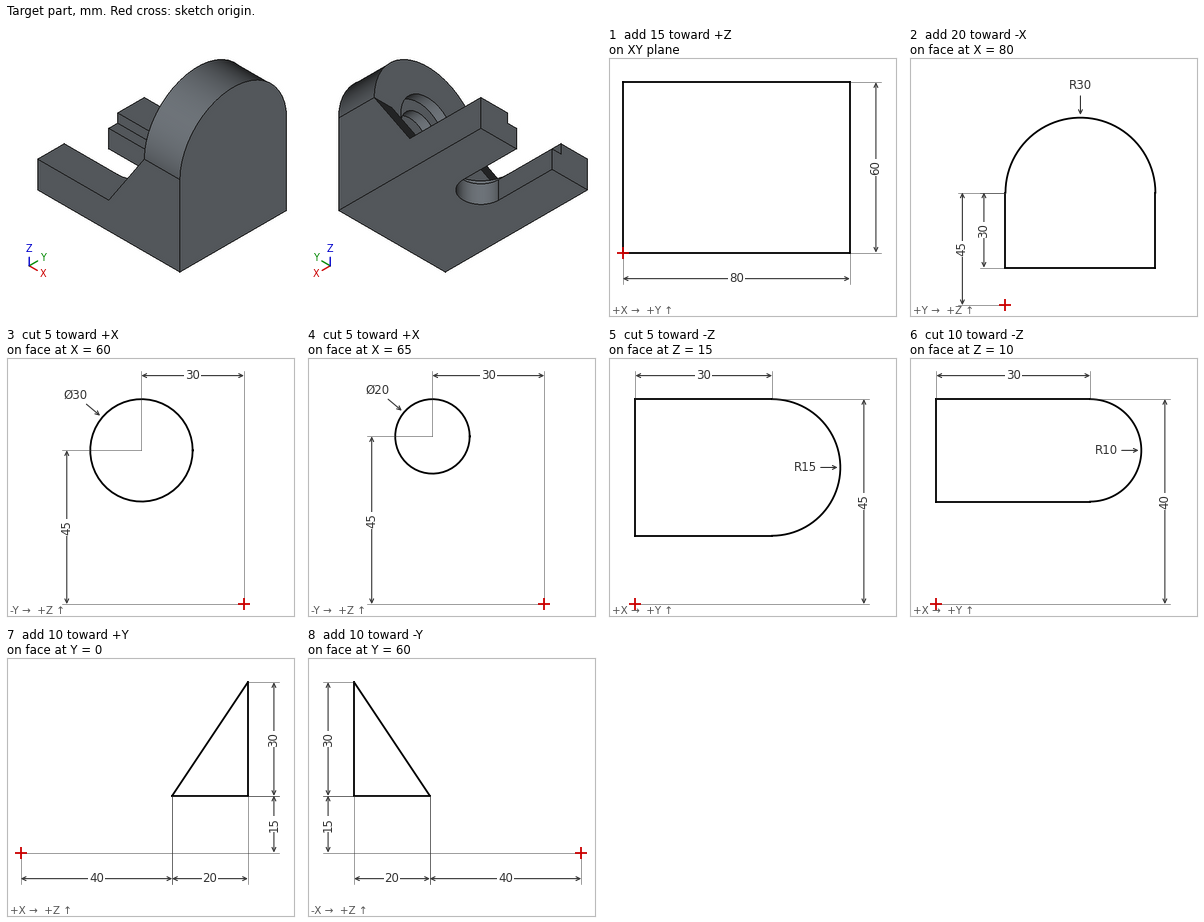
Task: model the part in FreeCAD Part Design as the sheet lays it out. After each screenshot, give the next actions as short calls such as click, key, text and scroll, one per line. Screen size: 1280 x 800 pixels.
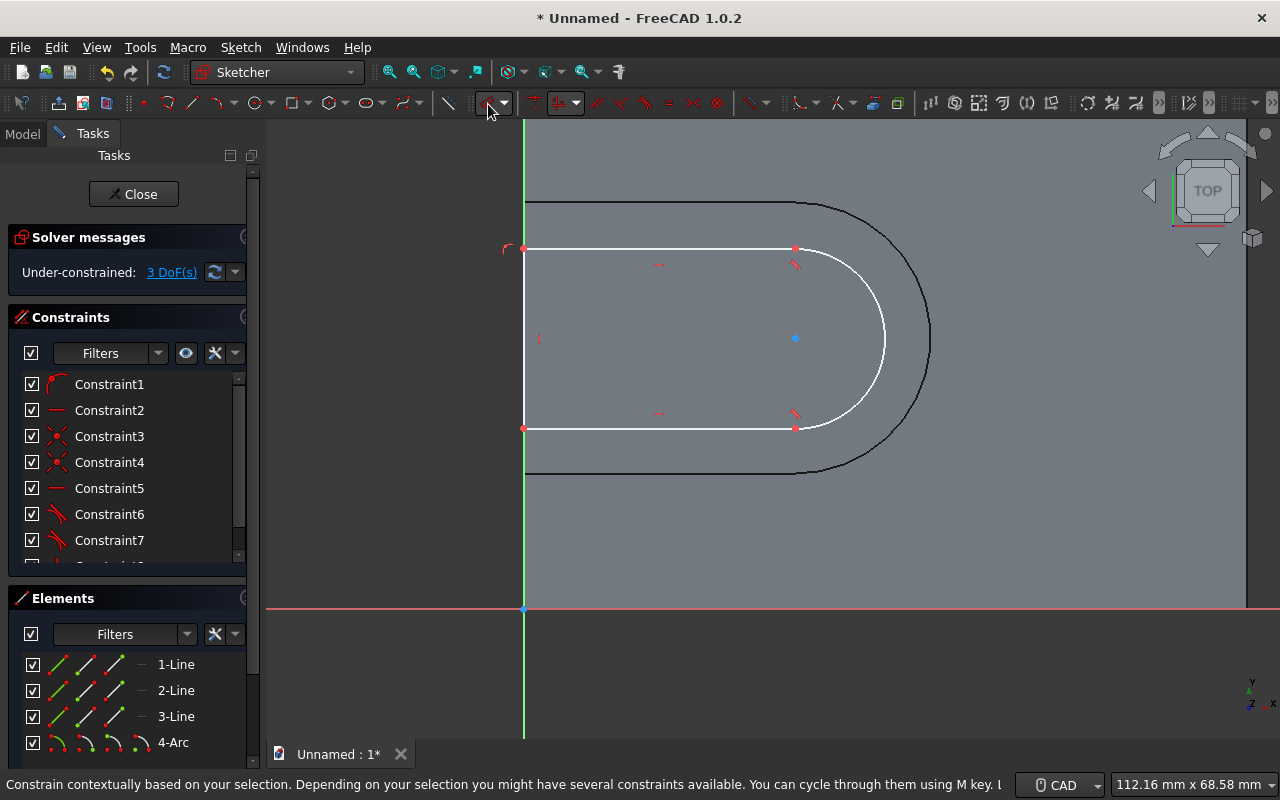
click(868, 392)
click(894, 411)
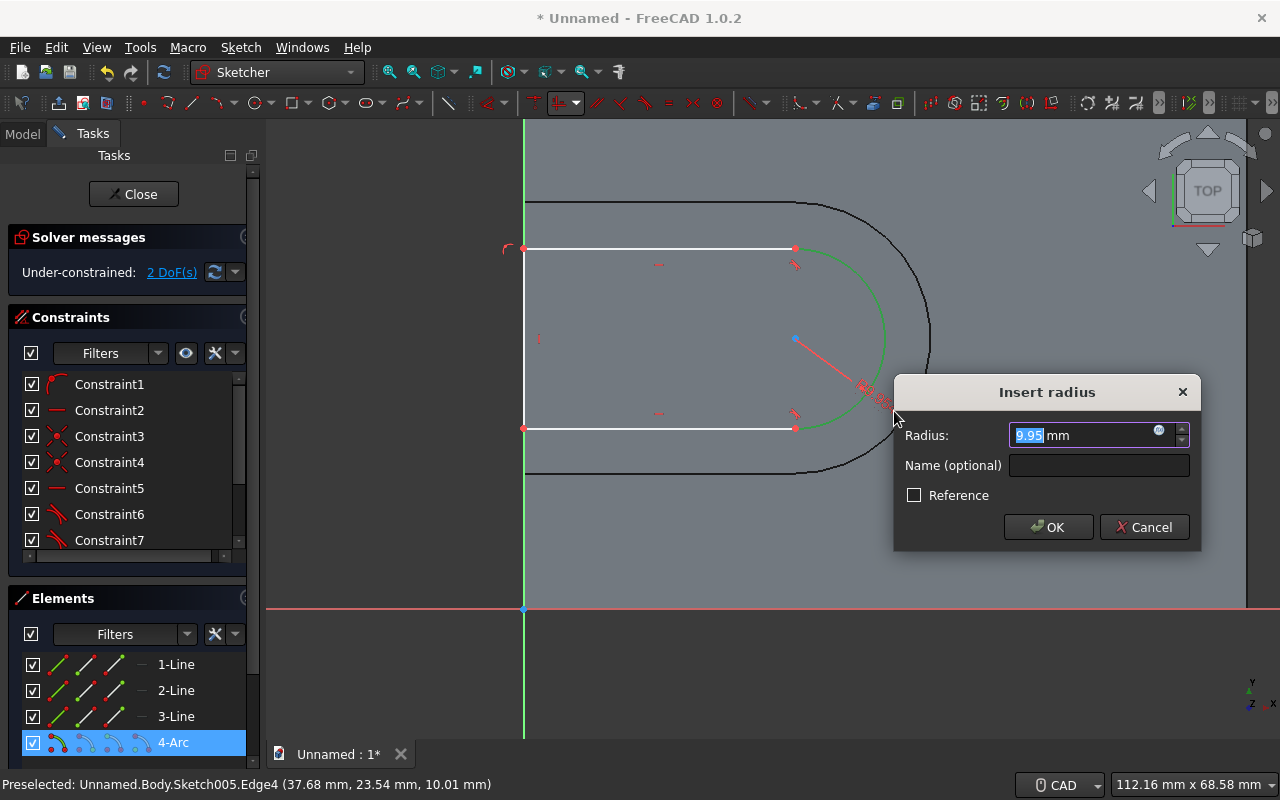
text(10)
key(Return)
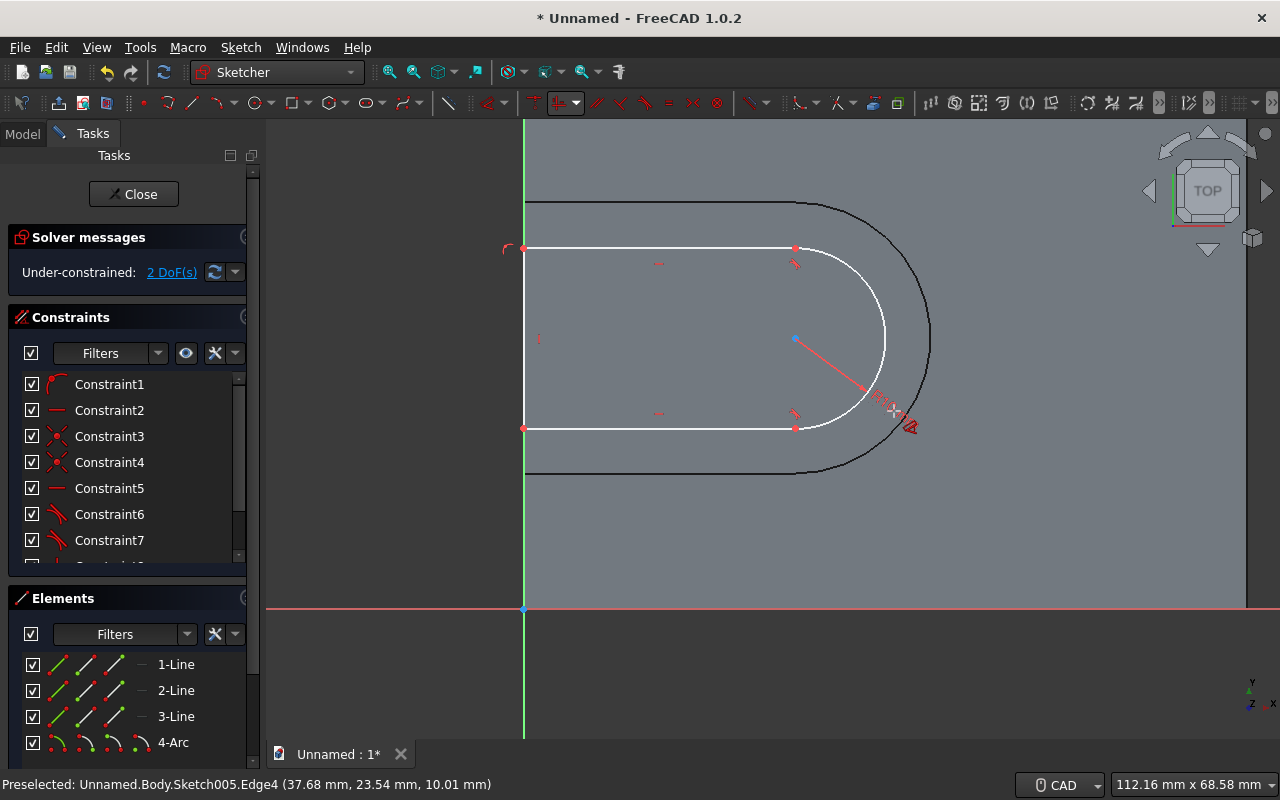
click(714, 248)
click(659, 214)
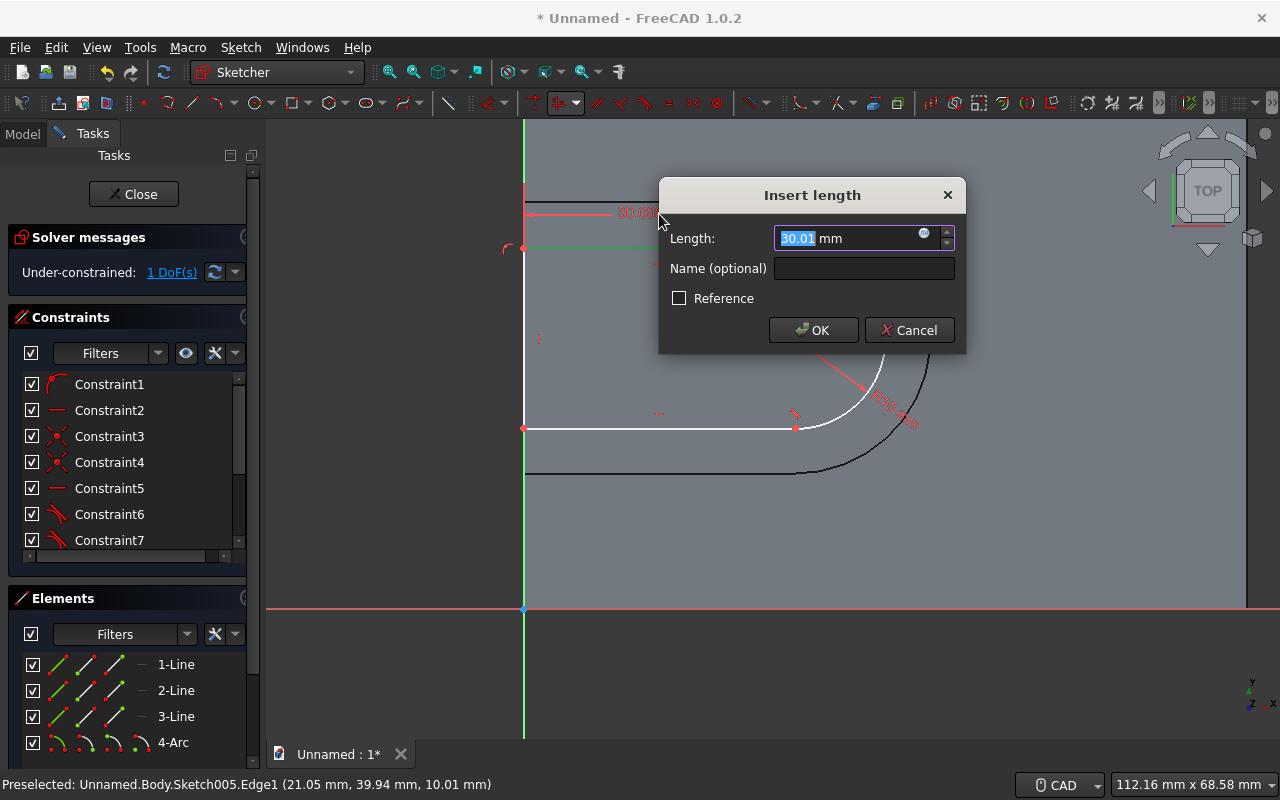
text(30)
key(Return)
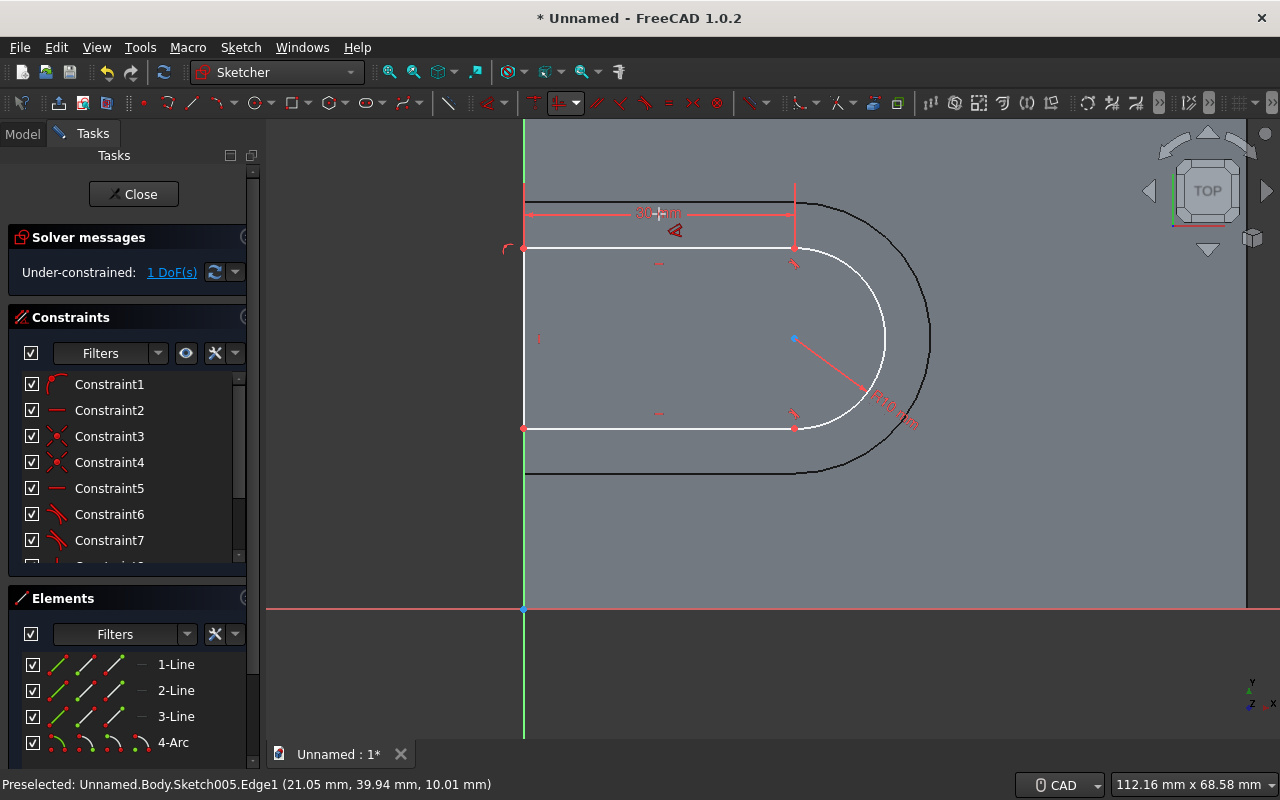
click(795, 248)
click(490, 429)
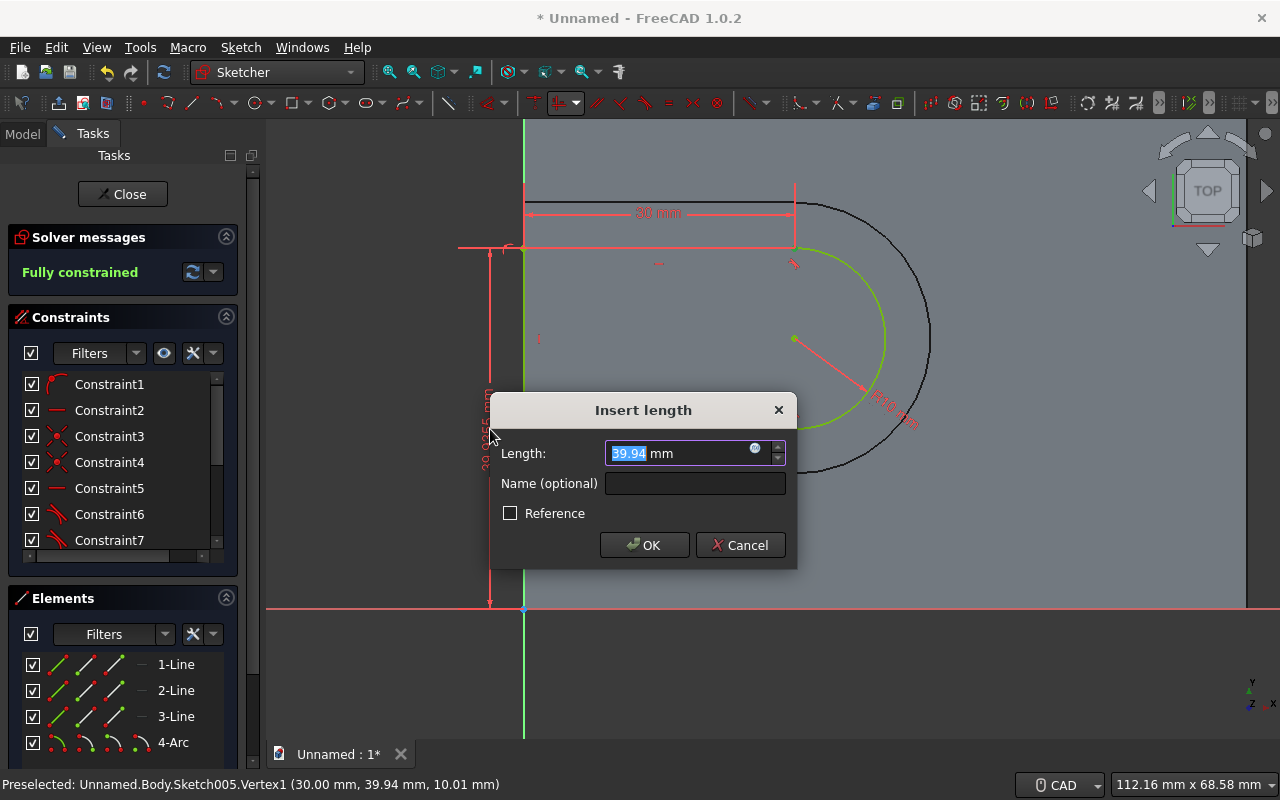
text(40)
key(Return)
key(Escape)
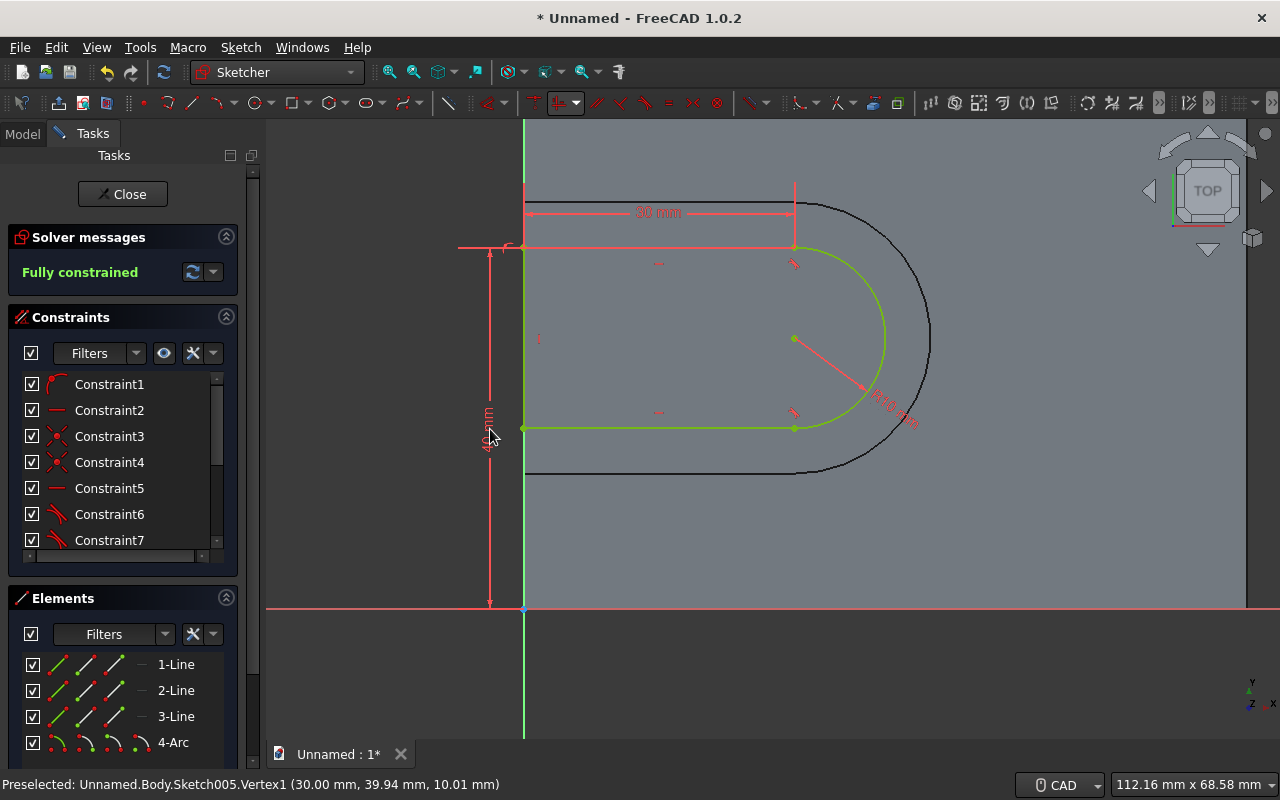
click(123, 194)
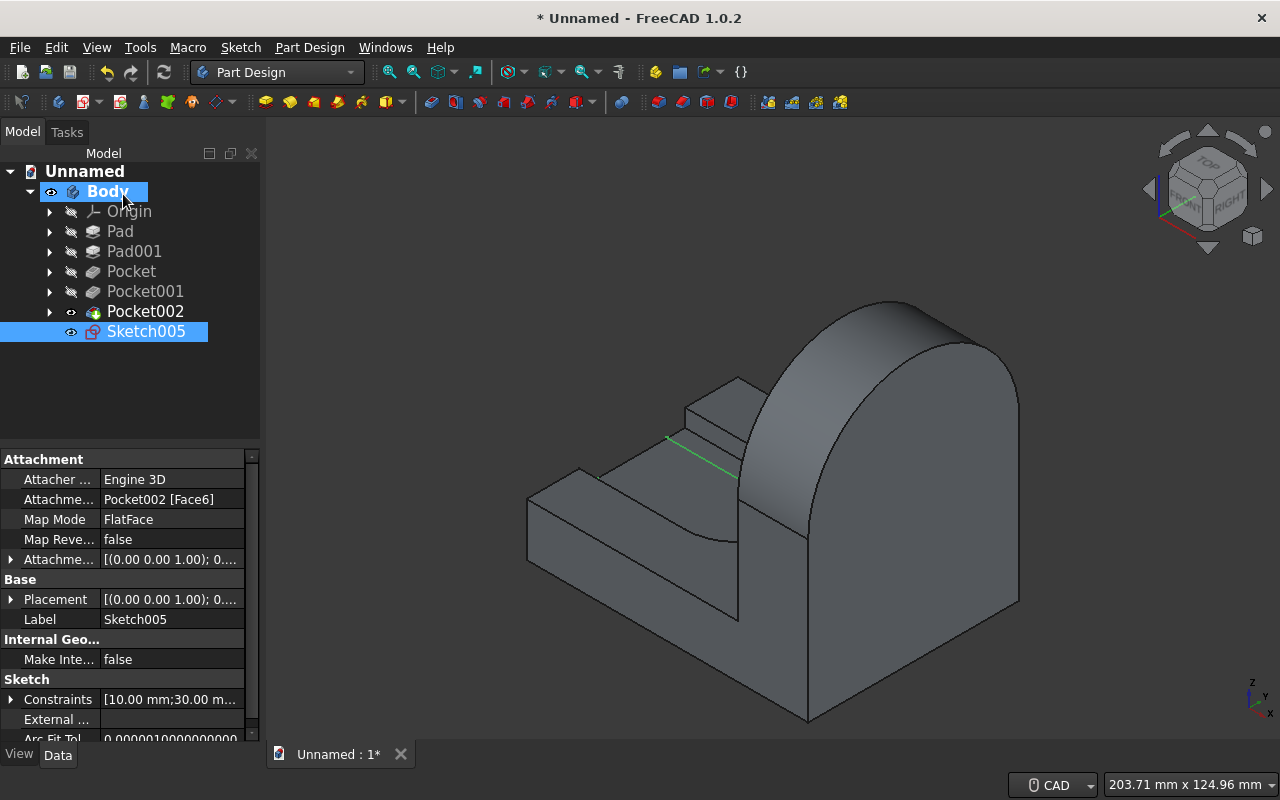
click(432, 102)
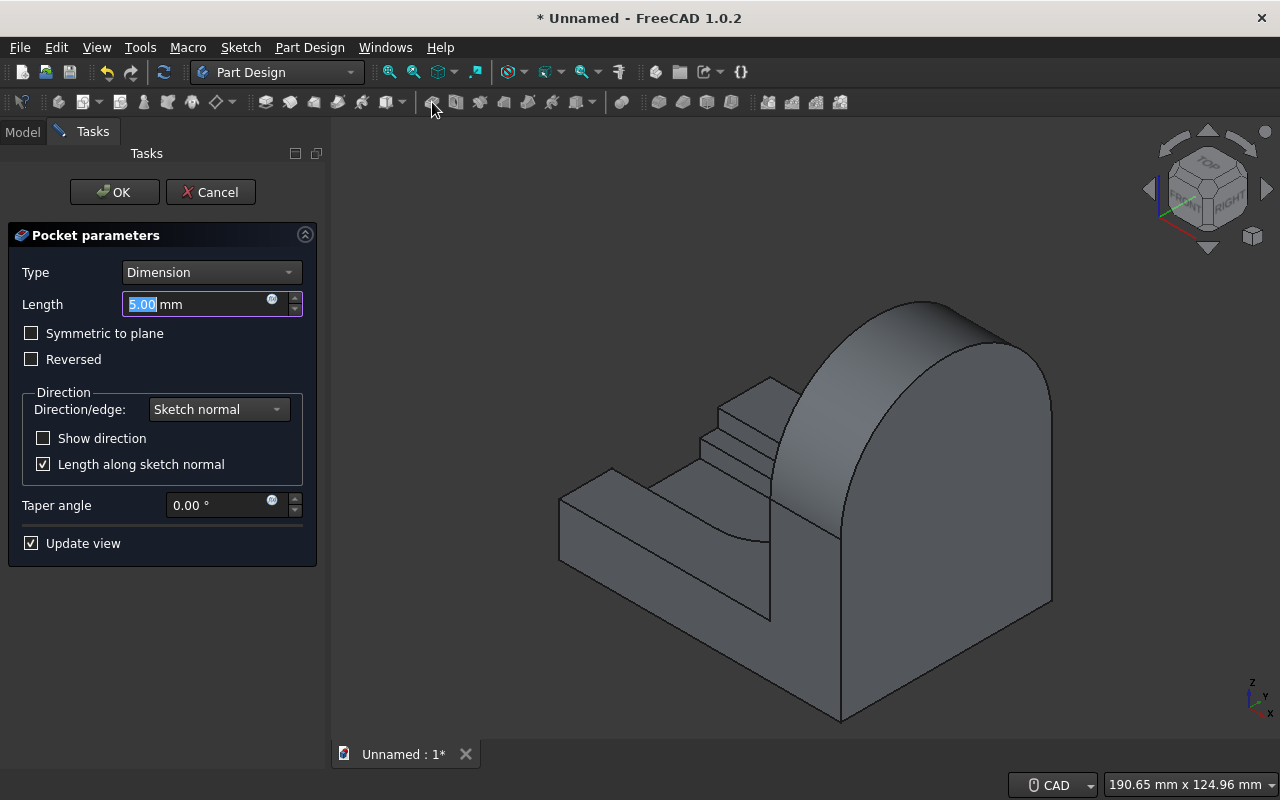
text(10)
key(Tab)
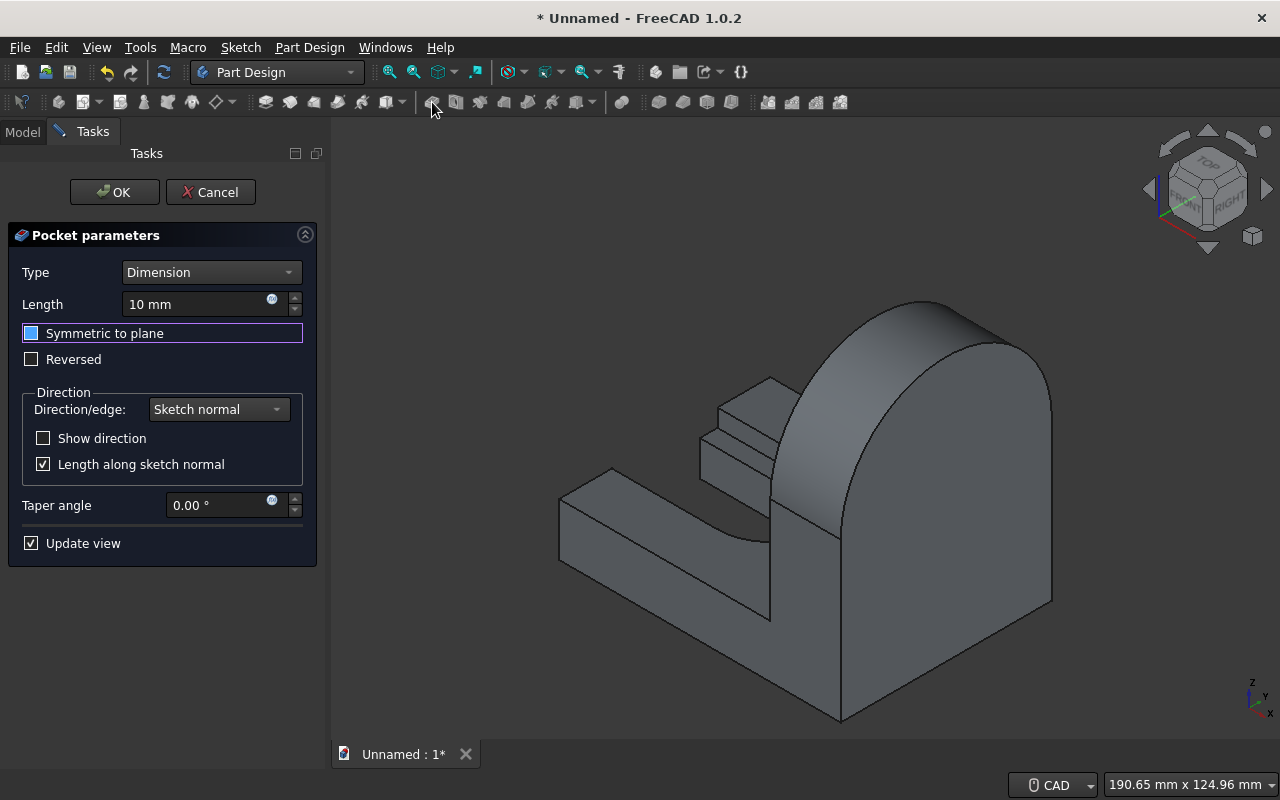
click(115, 192)